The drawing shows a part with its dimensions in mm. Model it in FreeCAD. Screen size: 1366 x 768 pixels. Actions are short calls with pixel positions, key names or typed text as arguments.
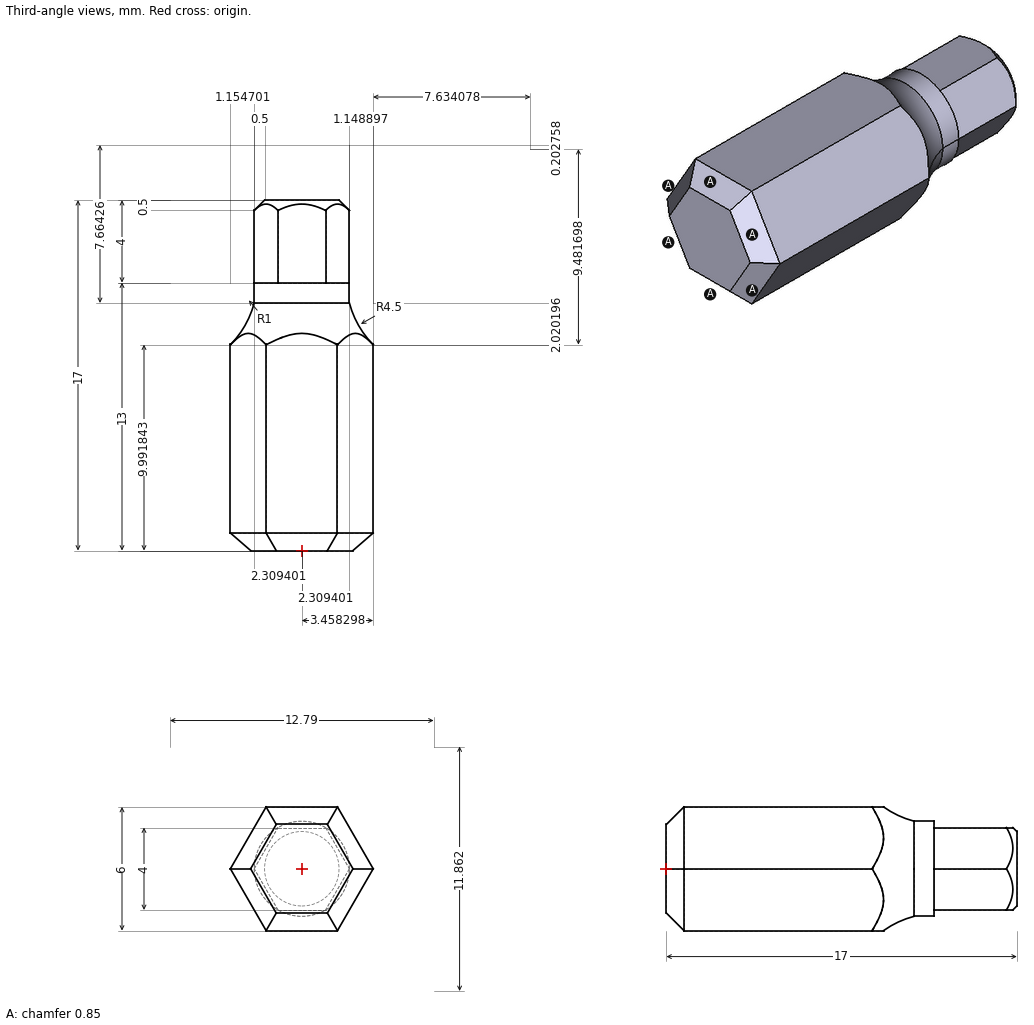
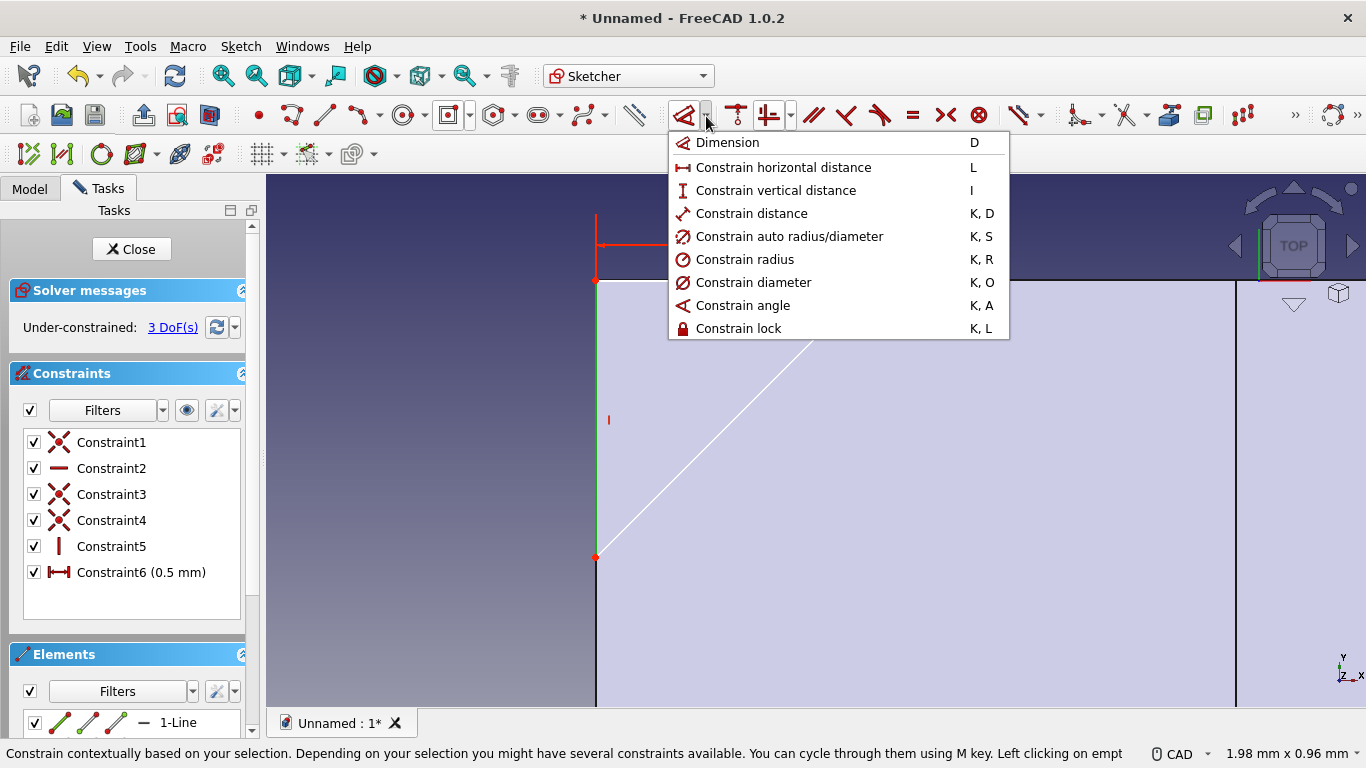
click(839, 190)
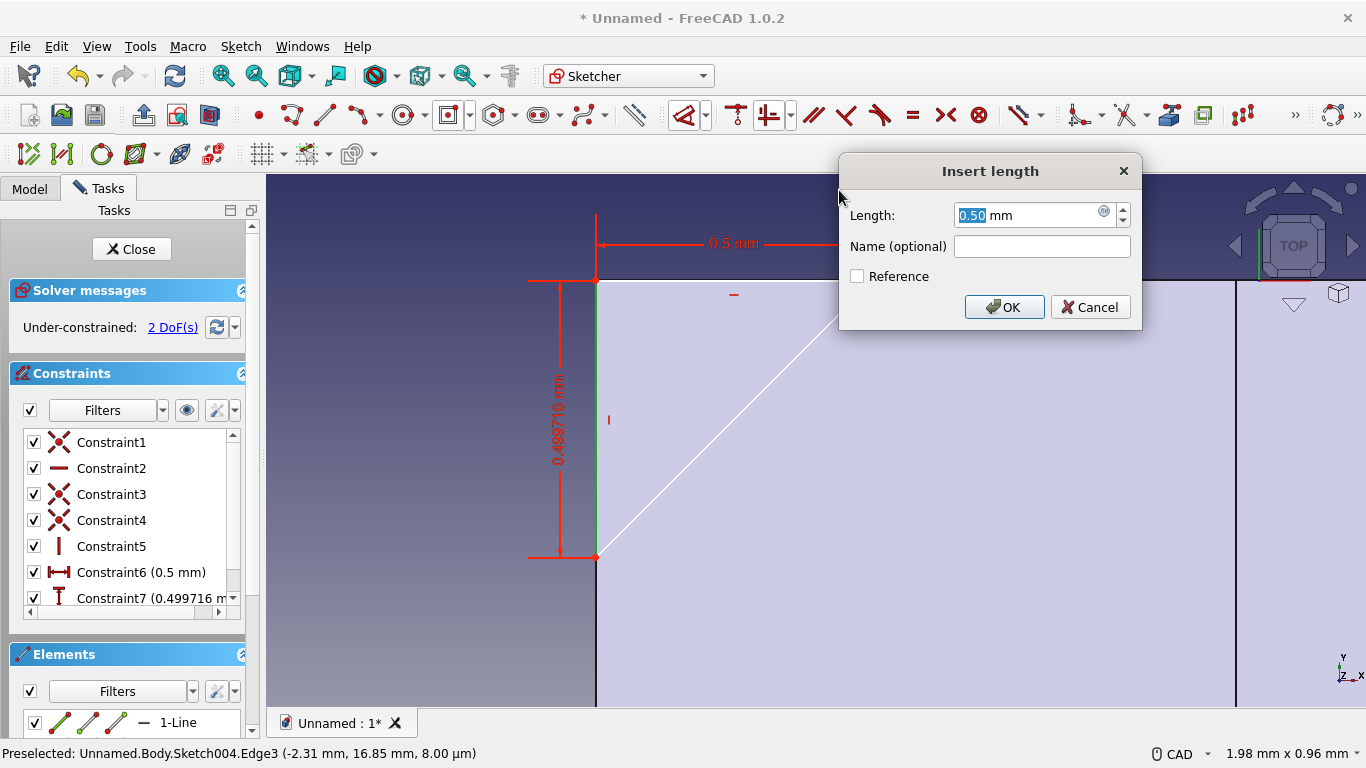
text(0.5)
key(Return)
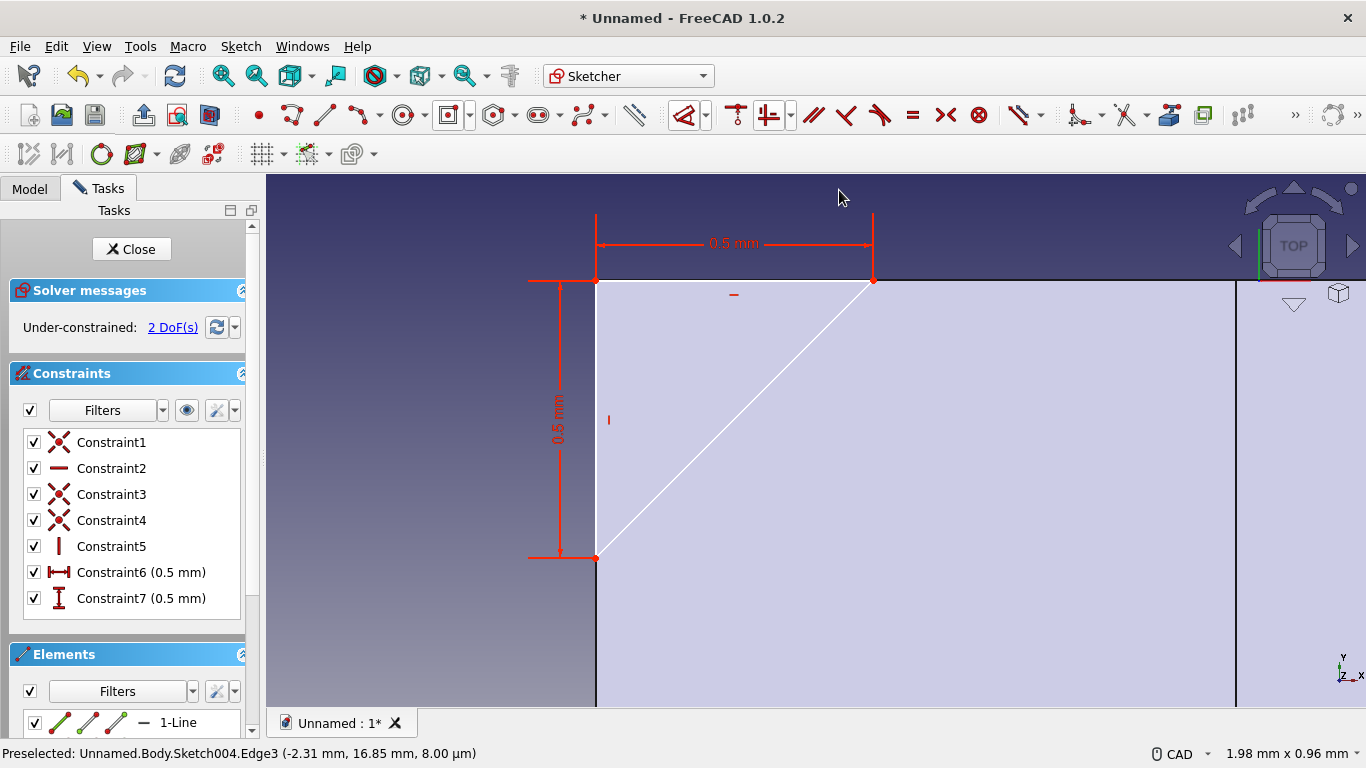
click(873, 281)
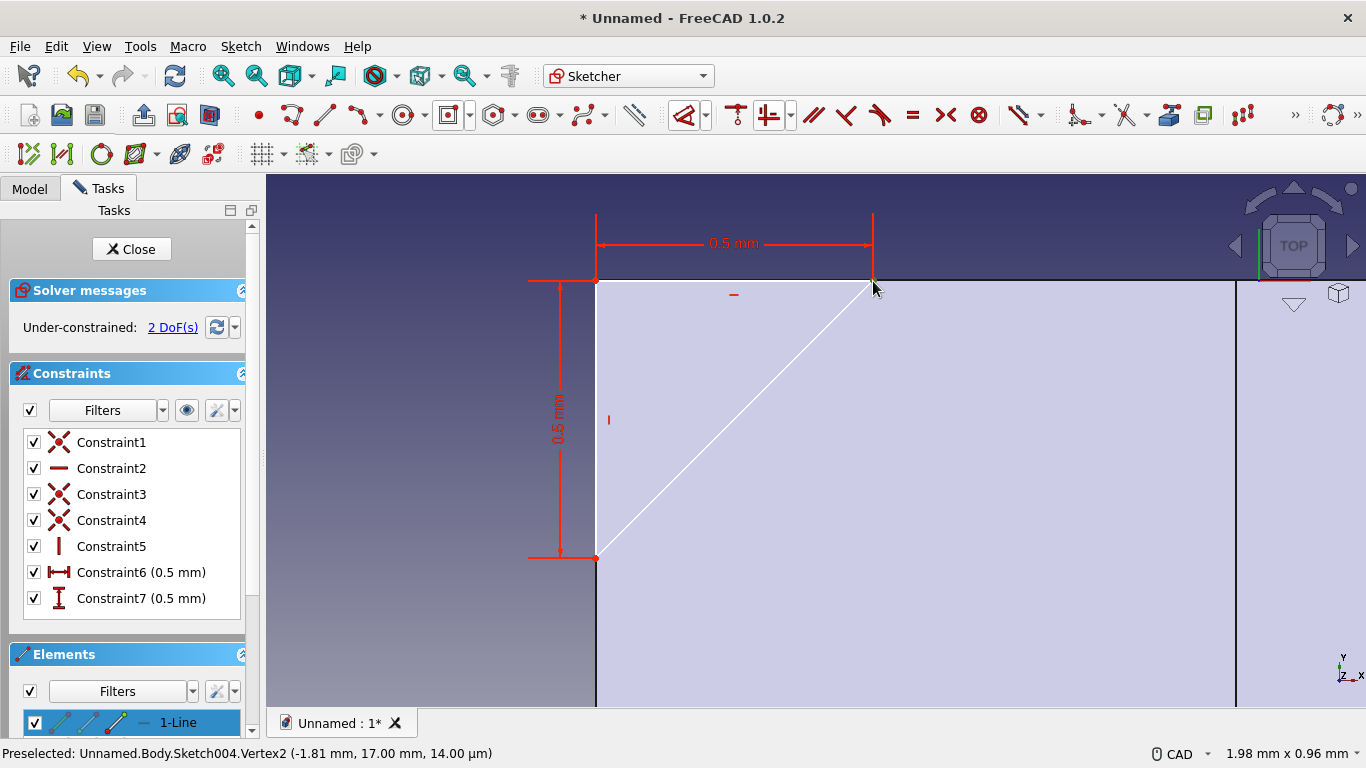
click(706, 116)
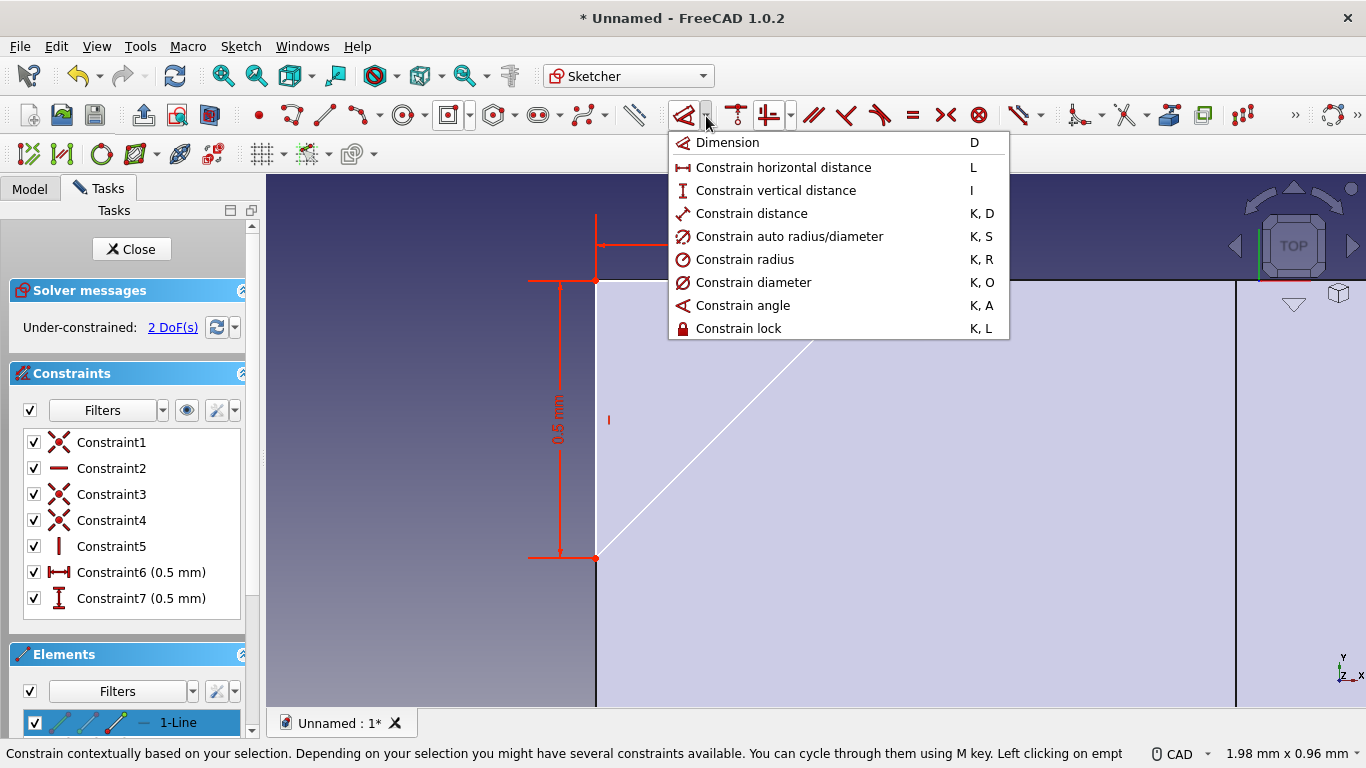
click(839, 190)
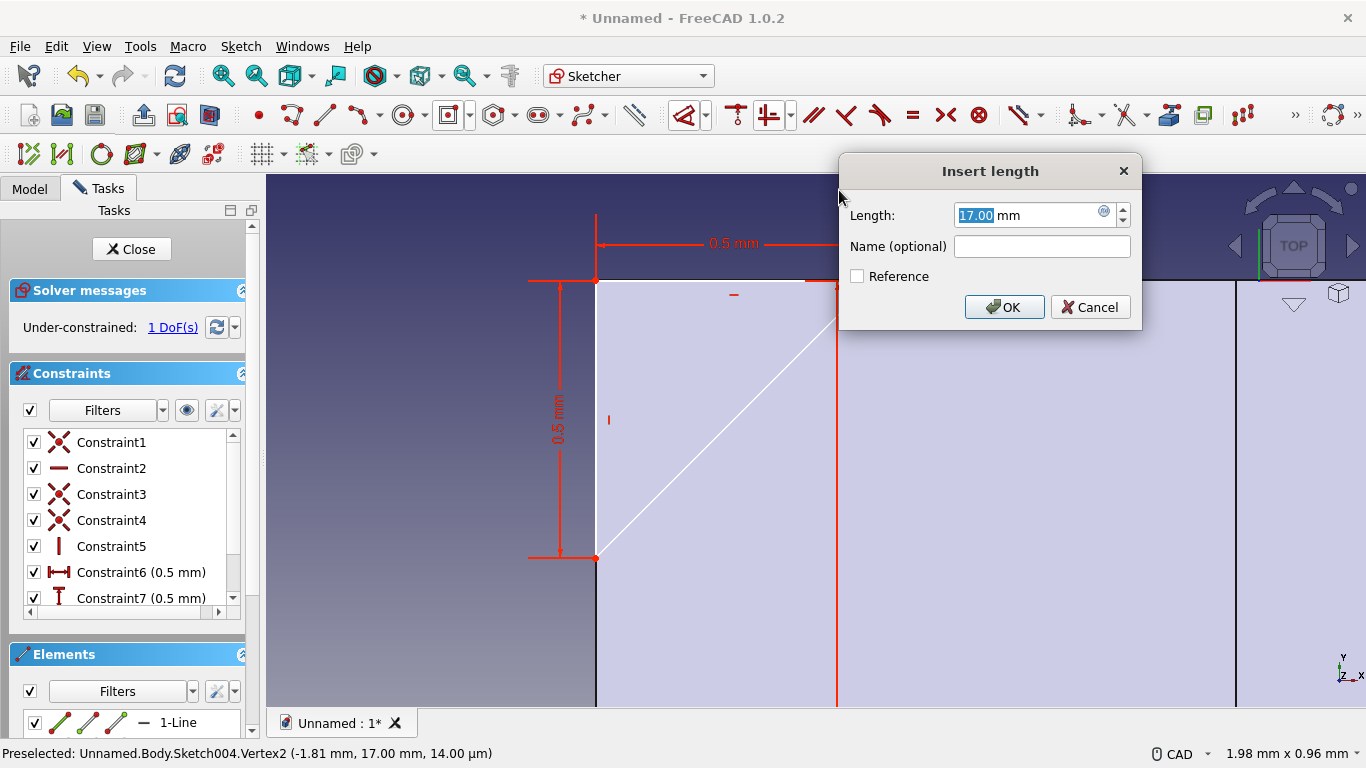
text(17)
key(Return)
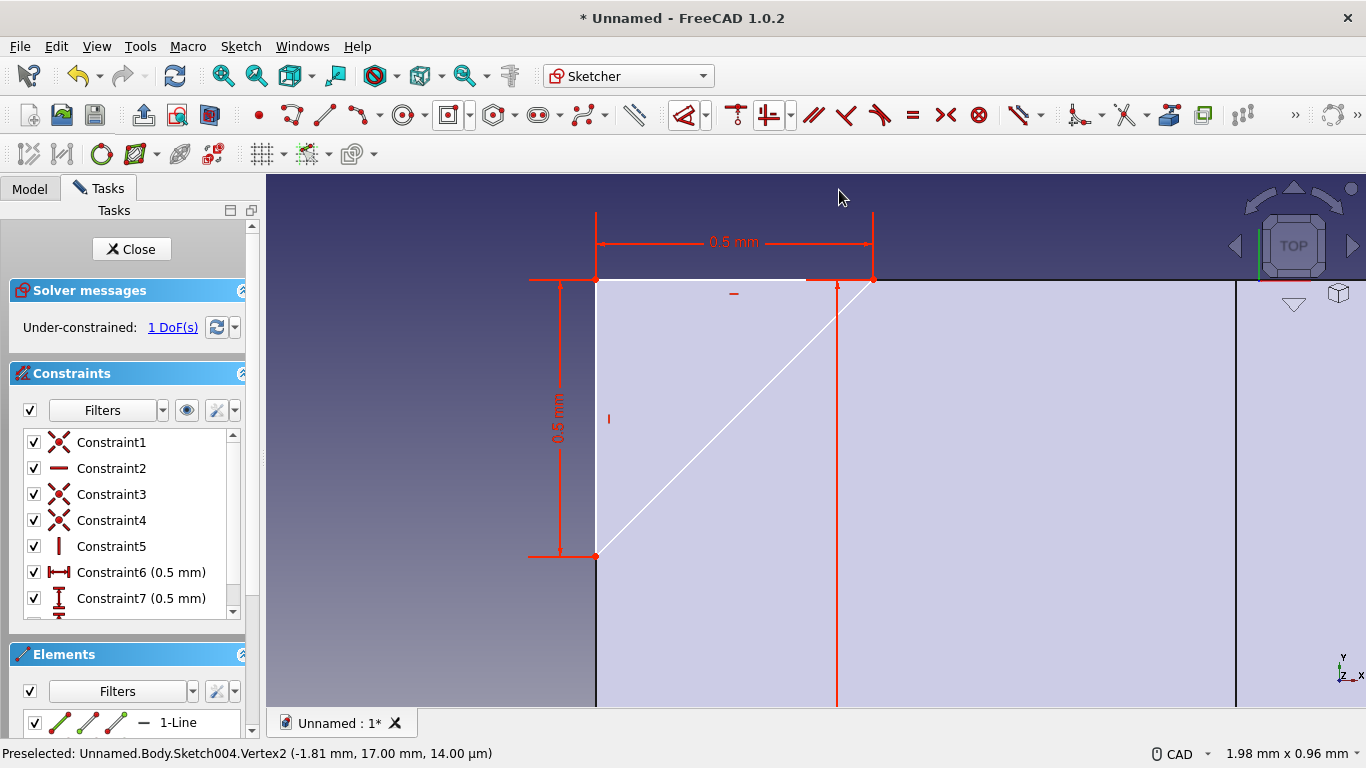
click(596, 557)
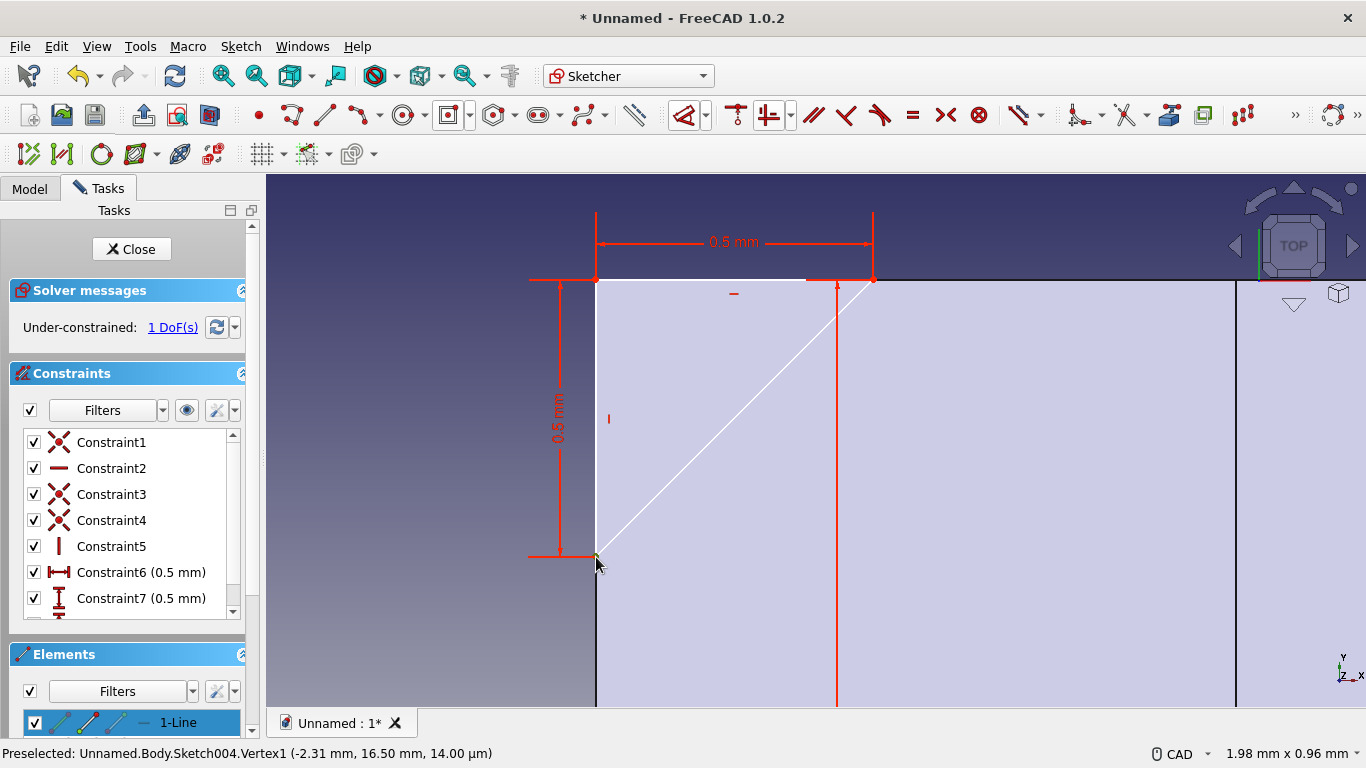
click(706, 116)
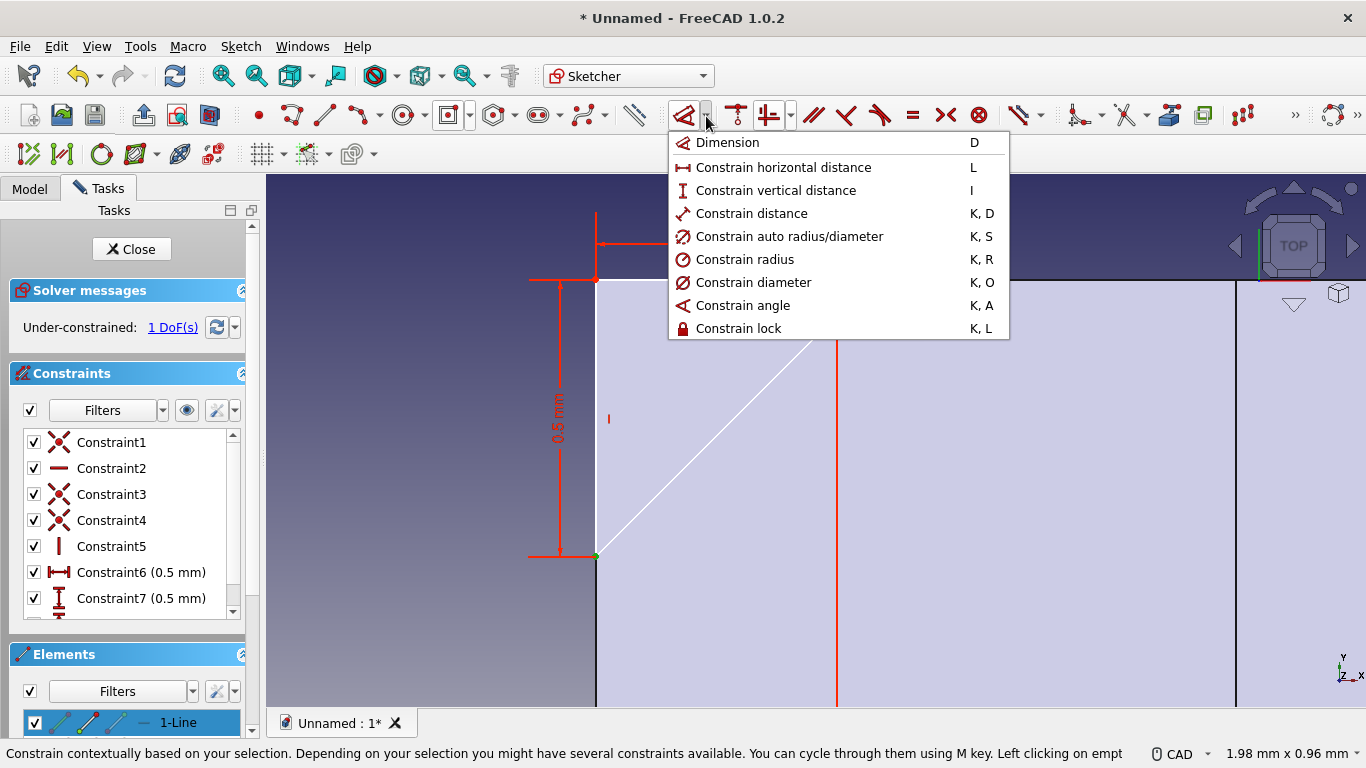
click(839, 168)